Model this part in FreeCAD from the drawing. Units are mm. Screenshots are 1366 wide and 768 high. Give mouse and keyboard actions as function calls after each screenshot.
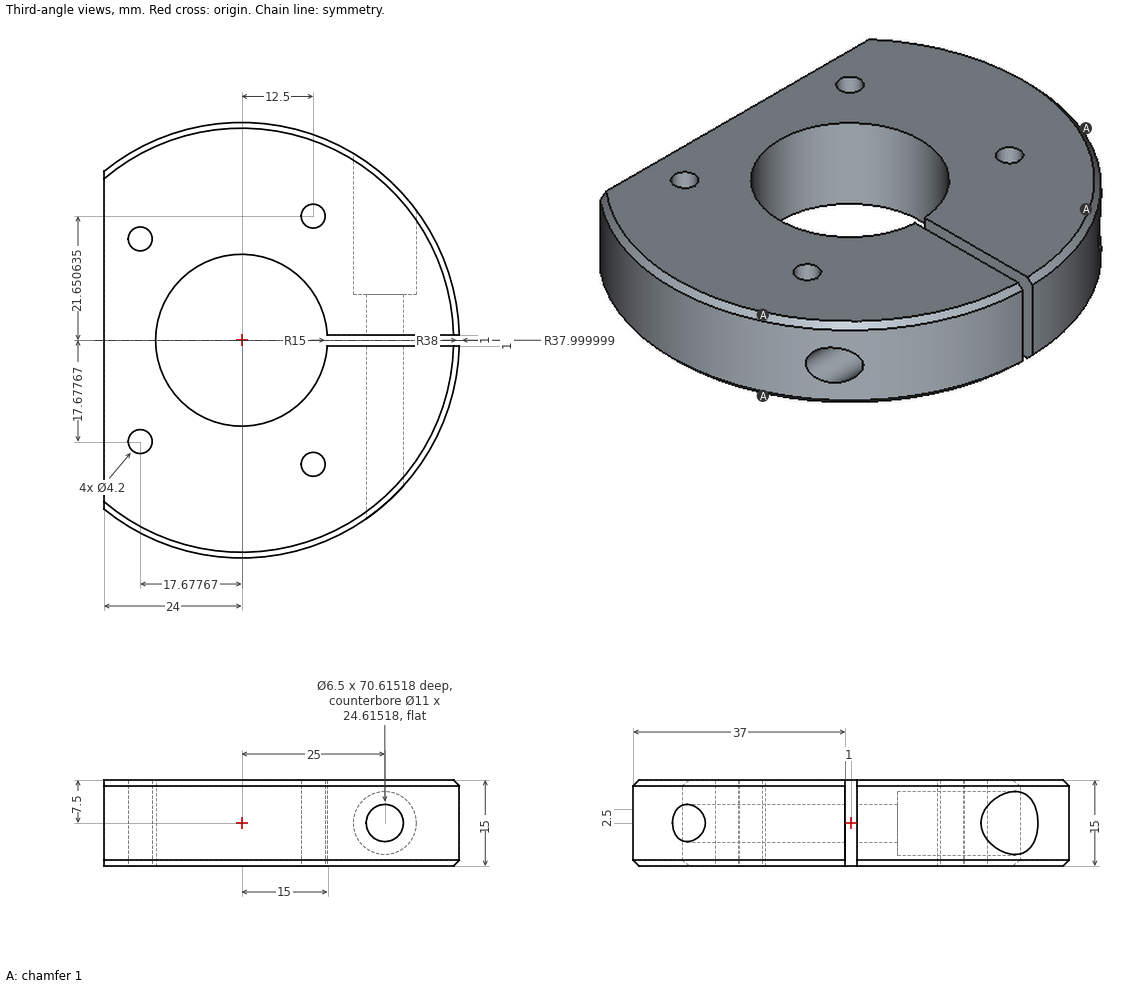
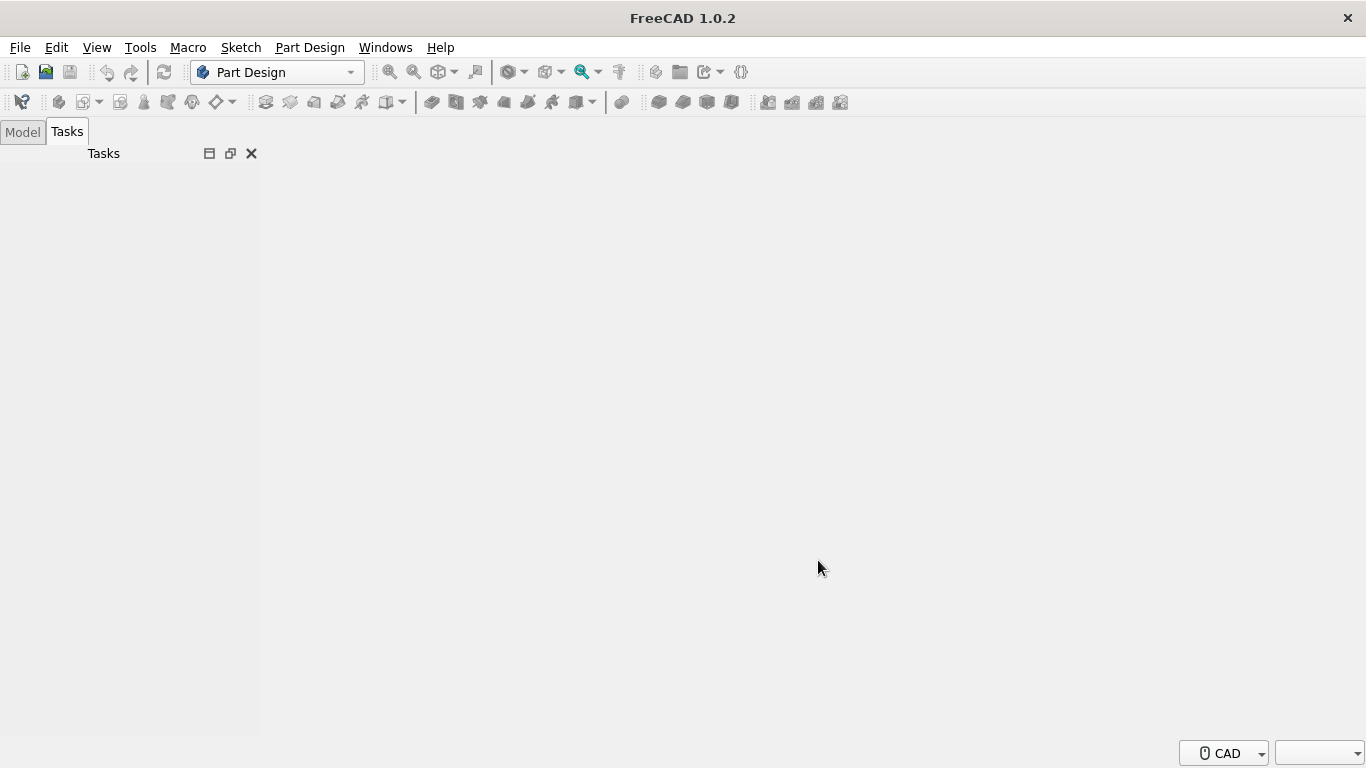
click(22, 72)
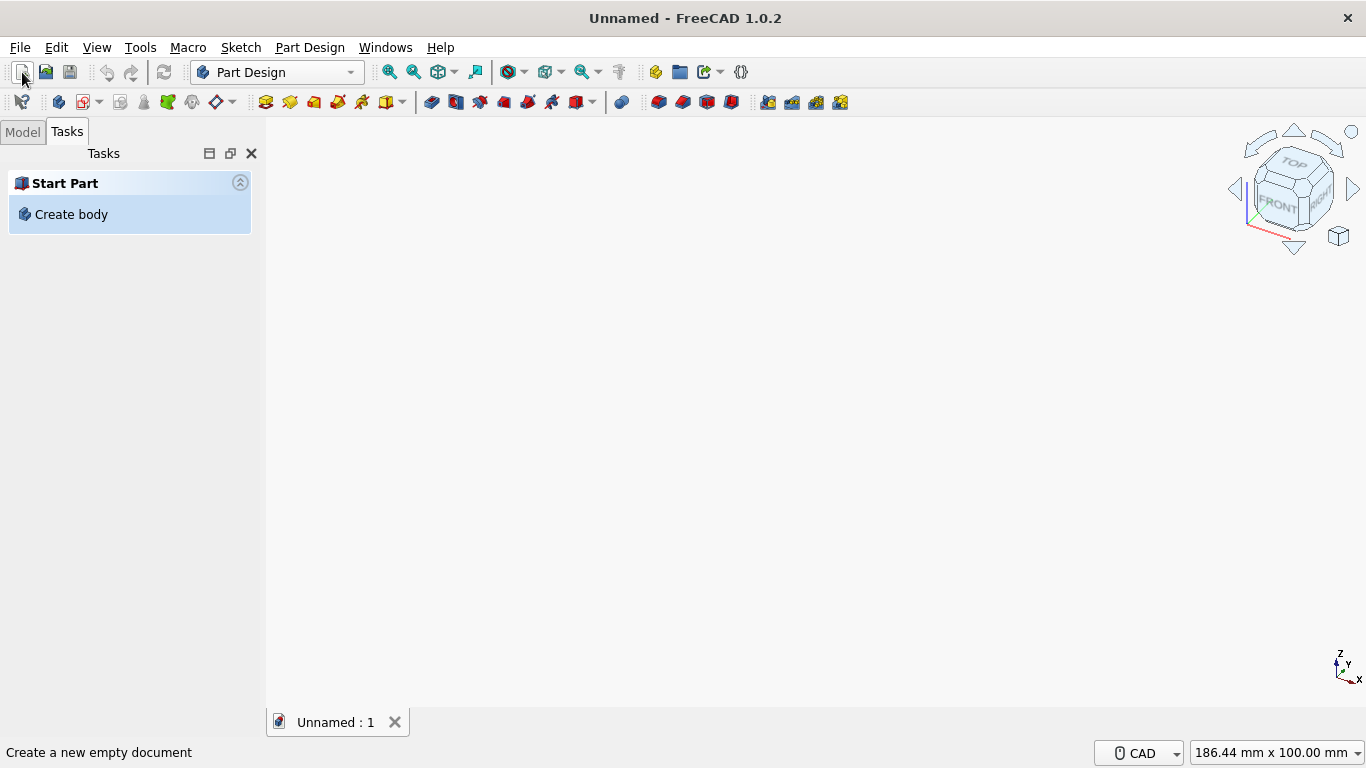
click(60, 102)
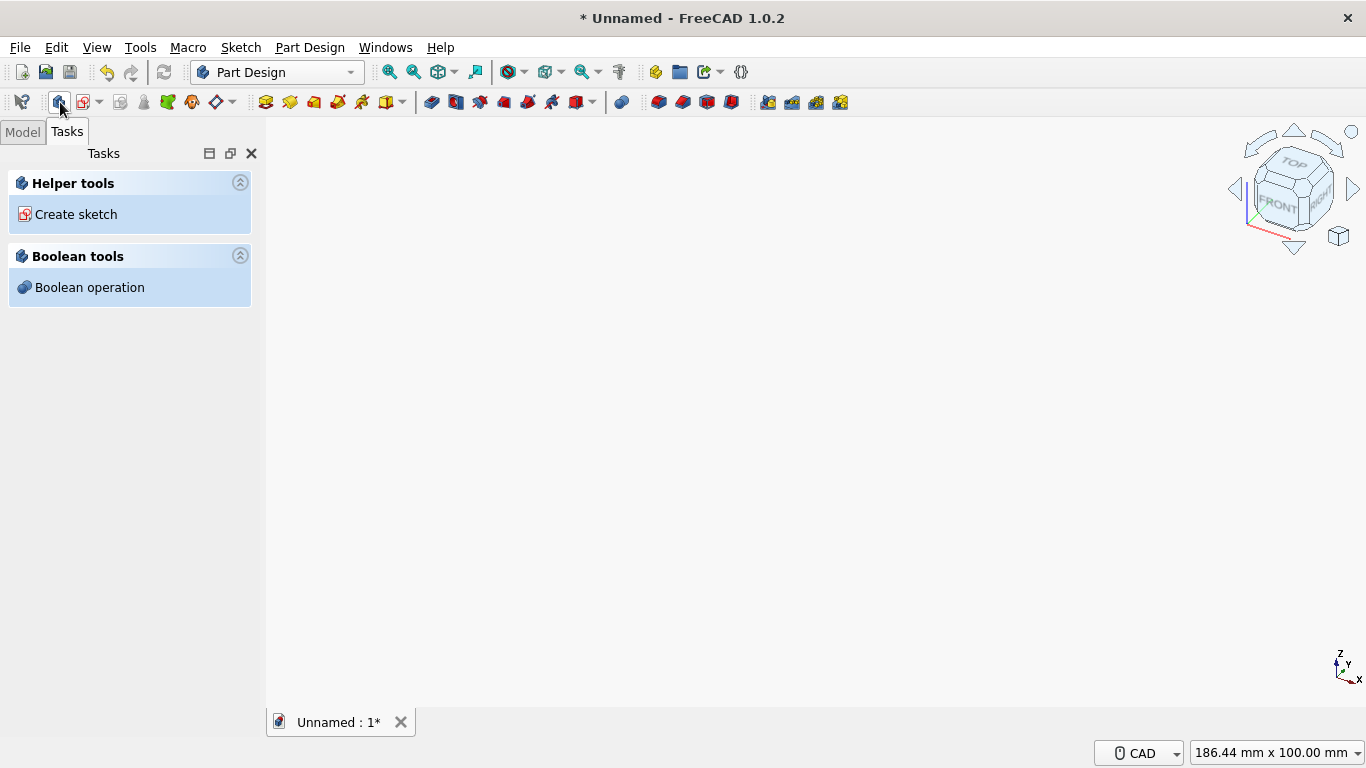
click(23, 131)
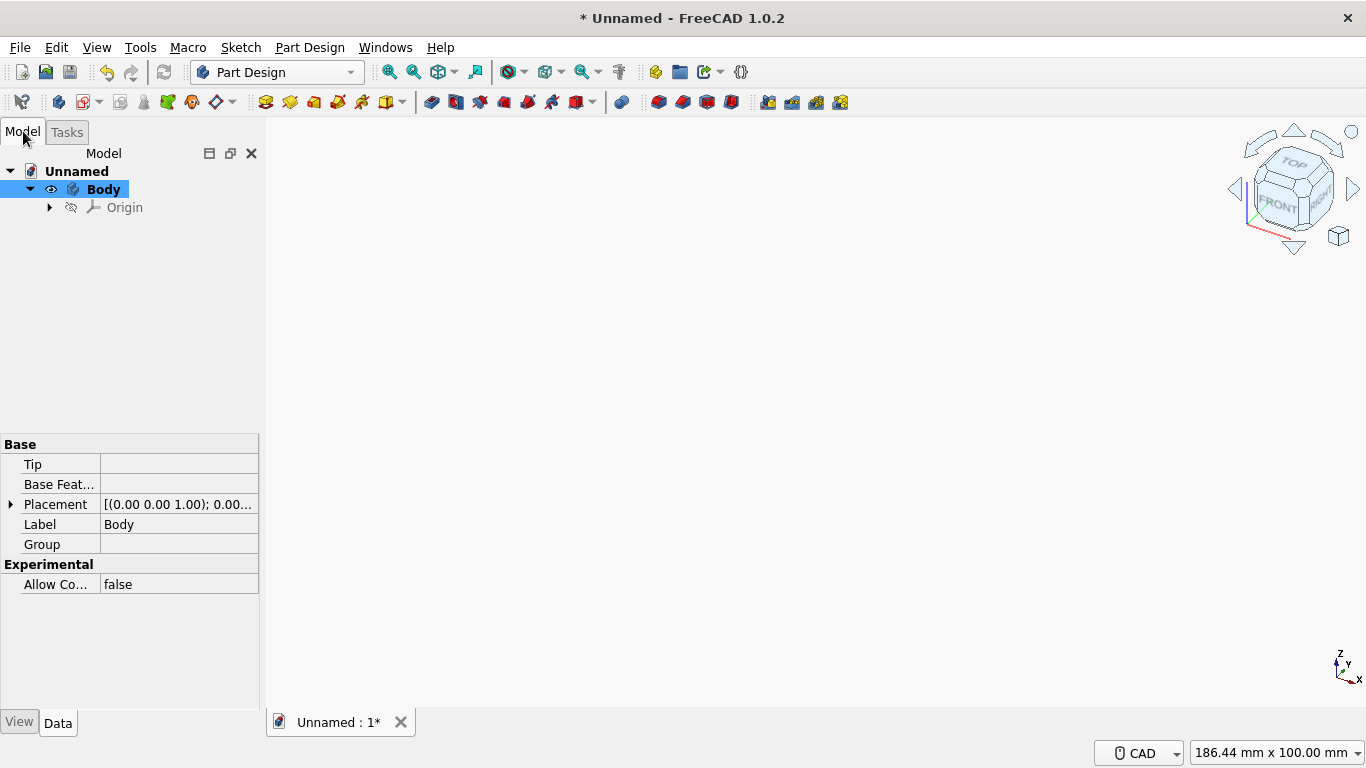
click(50, 207)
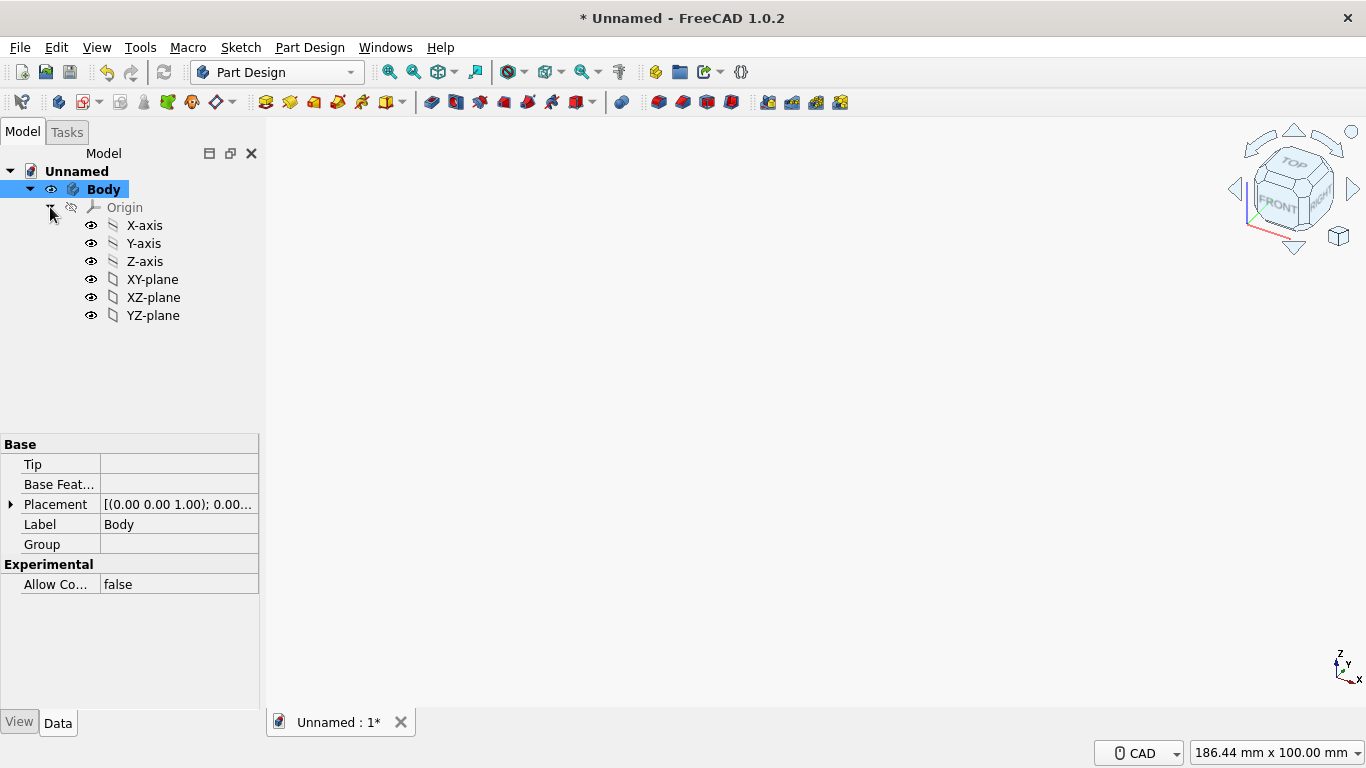
click(136, 279)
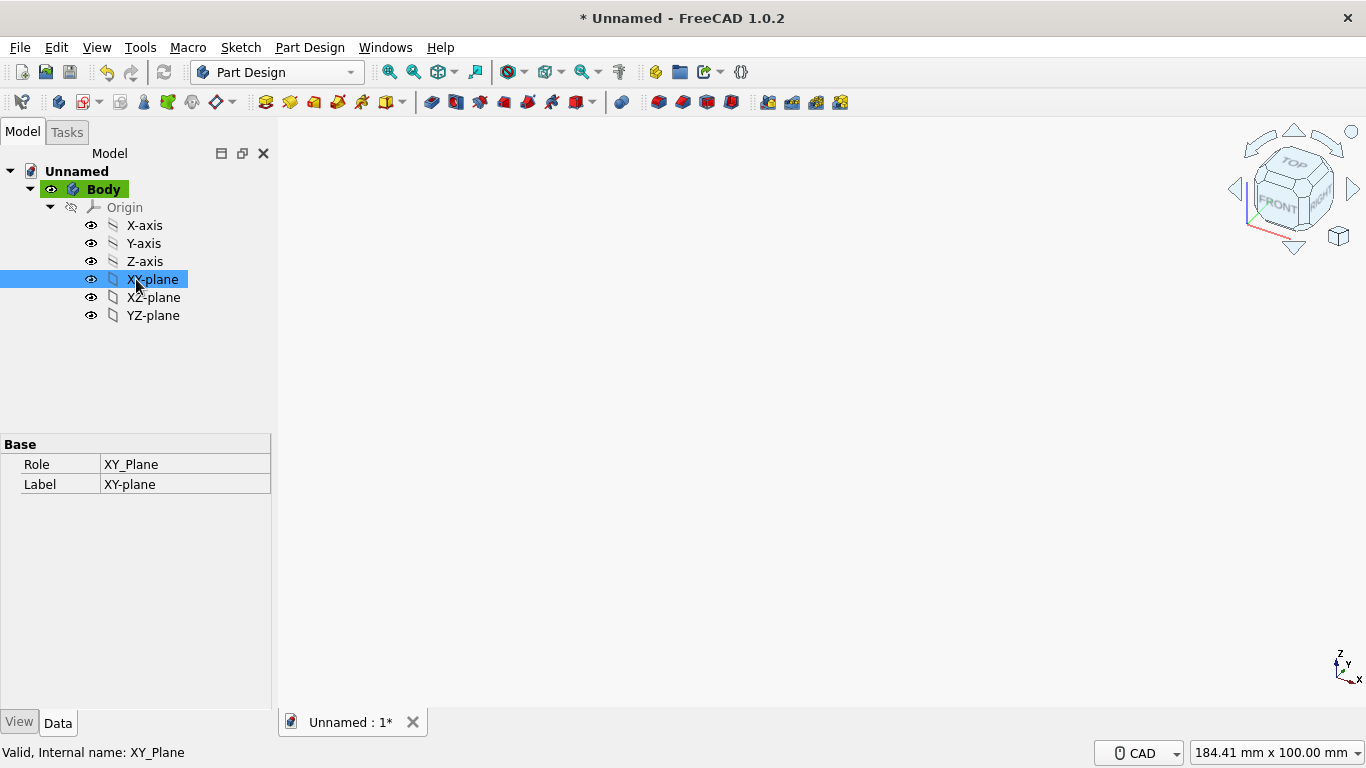
click(216, 102)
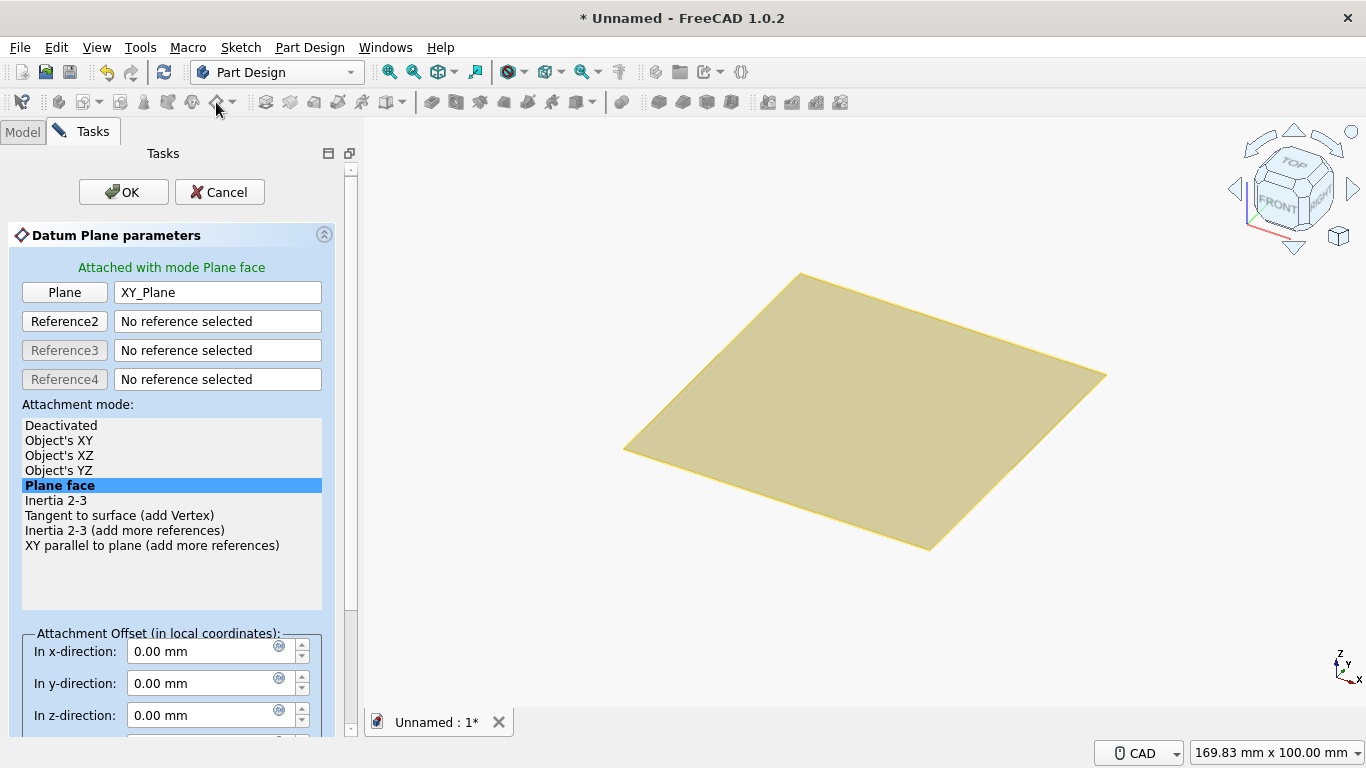
triple_click(210, 715)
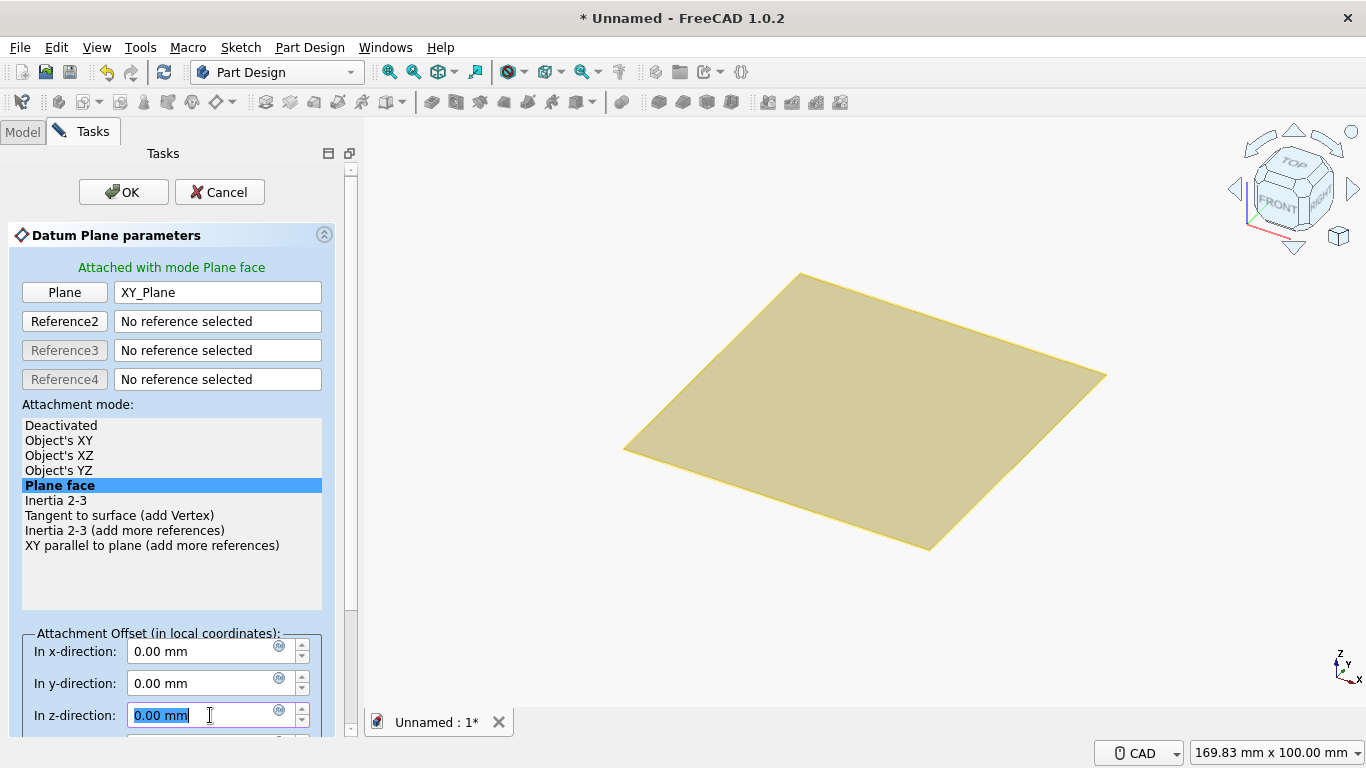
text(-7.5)
key(Tab)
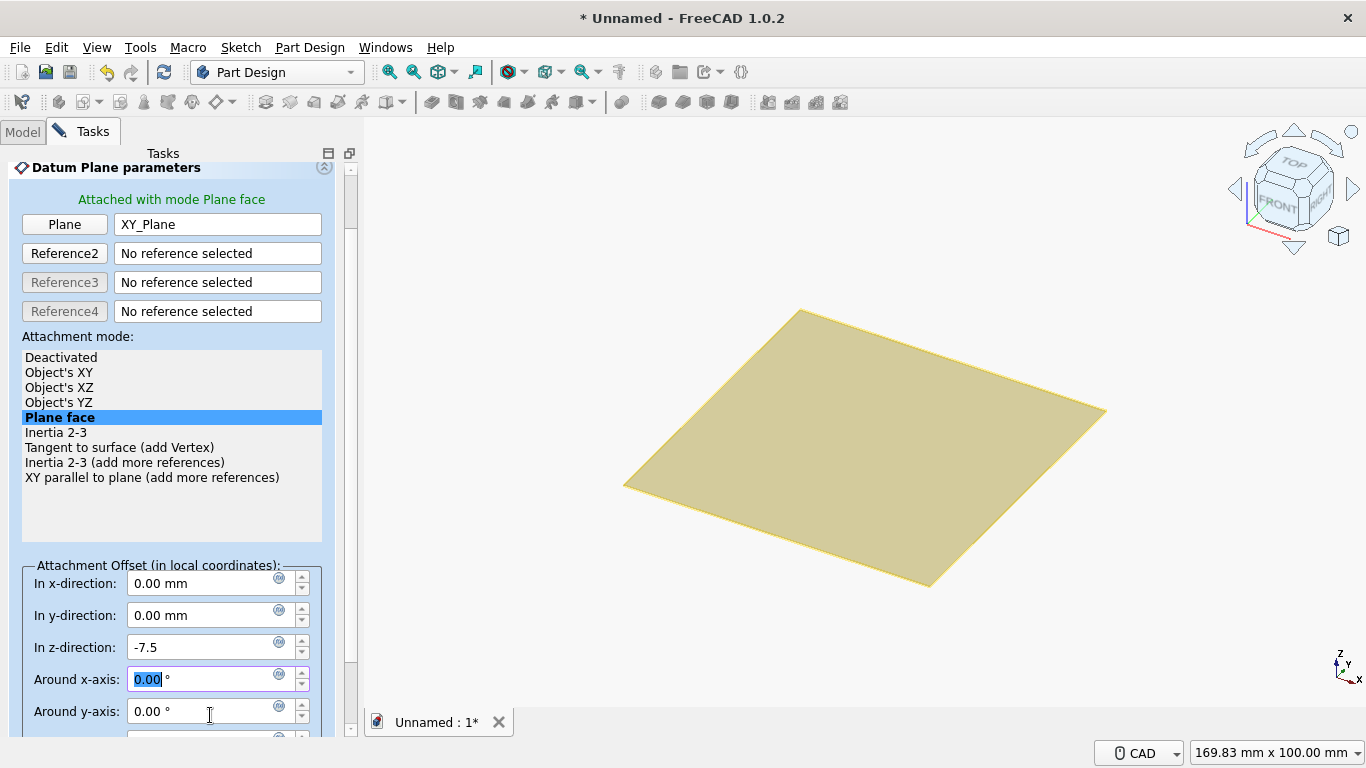
scroll(351, 450, up, 2)